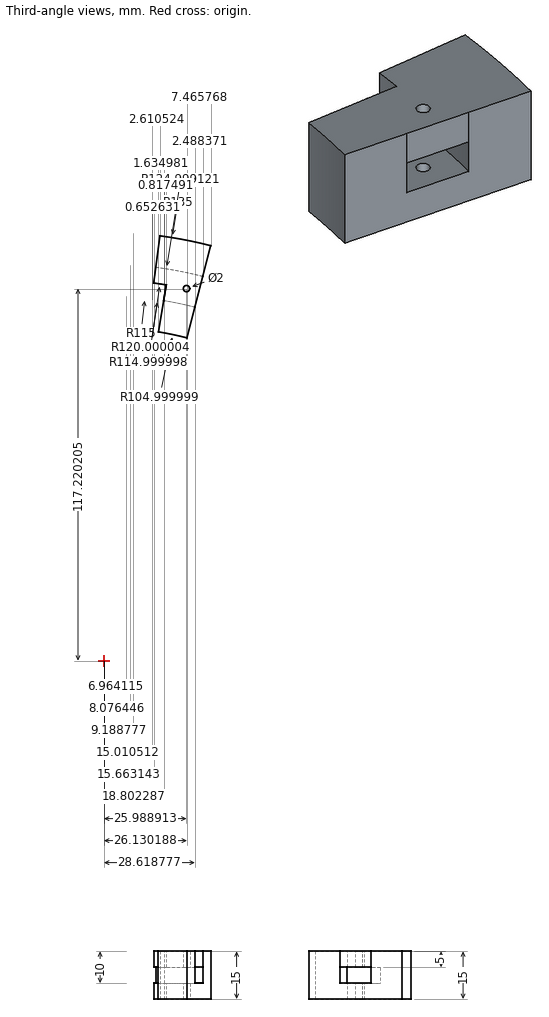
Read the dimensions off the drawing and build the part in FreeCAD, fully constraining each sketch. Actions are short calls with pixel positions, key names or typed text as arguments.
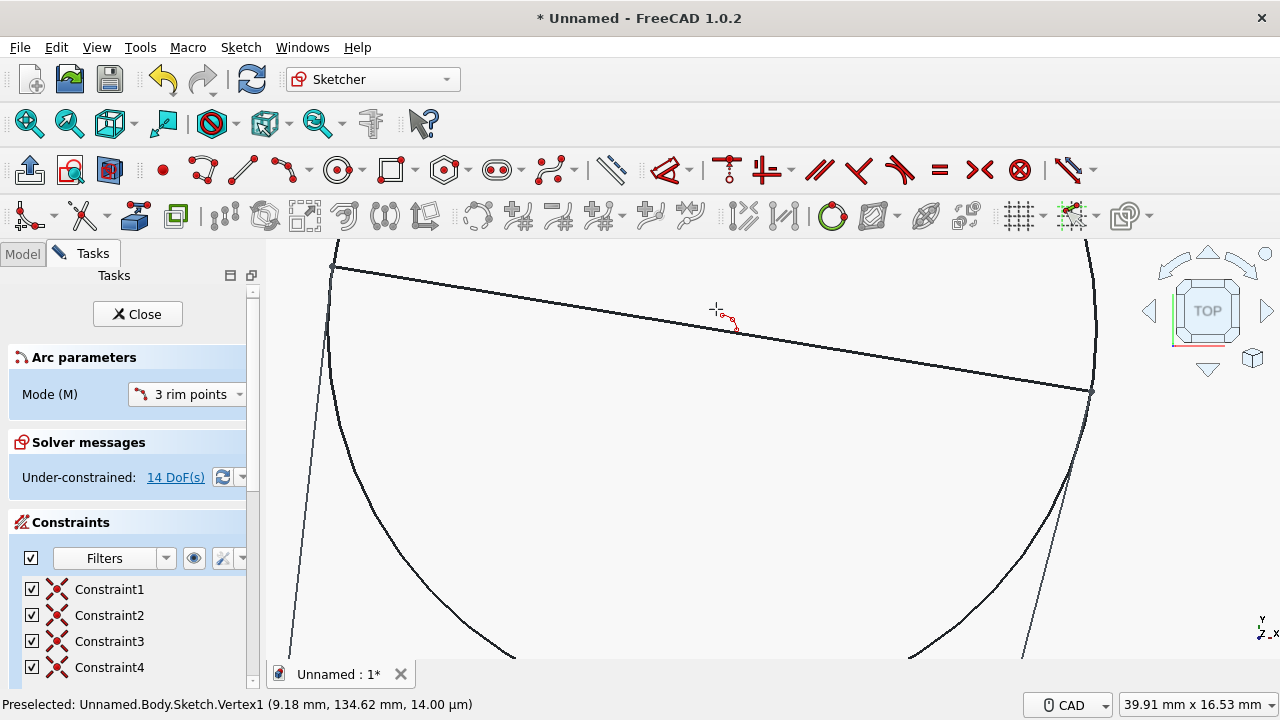
click(714, 308)
key(Escape)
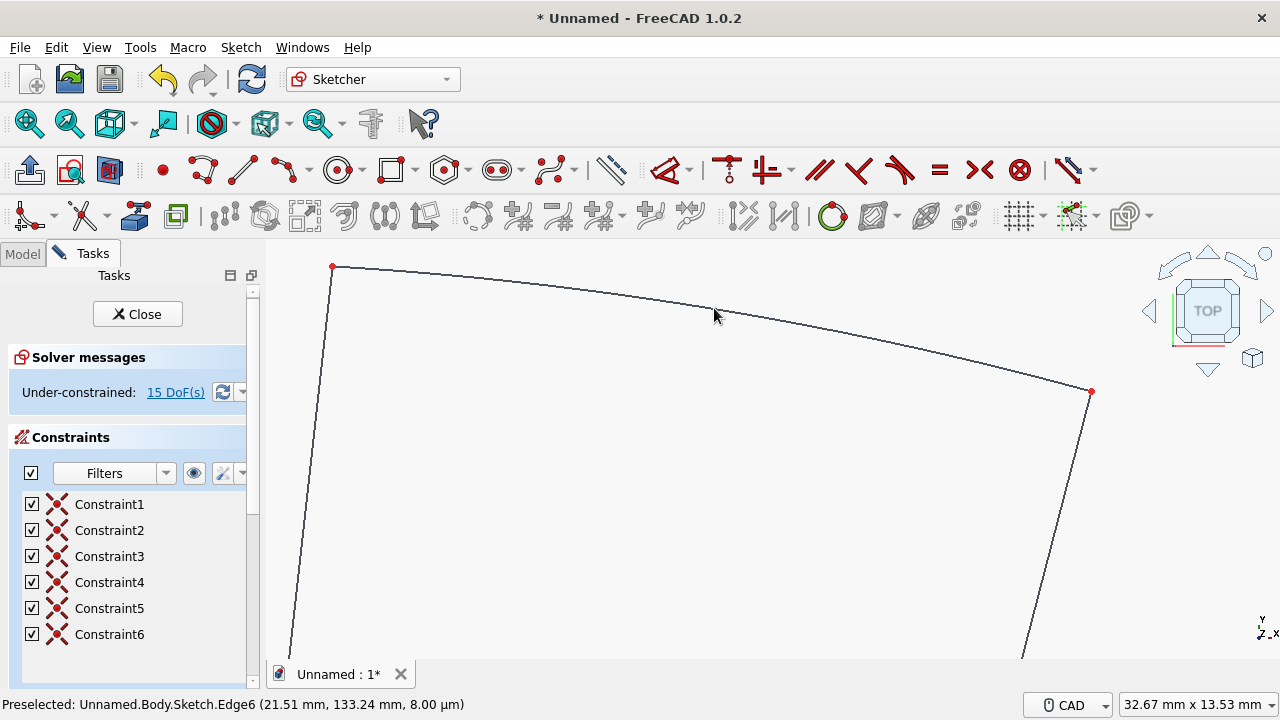
scroll(713, 342, down, 7)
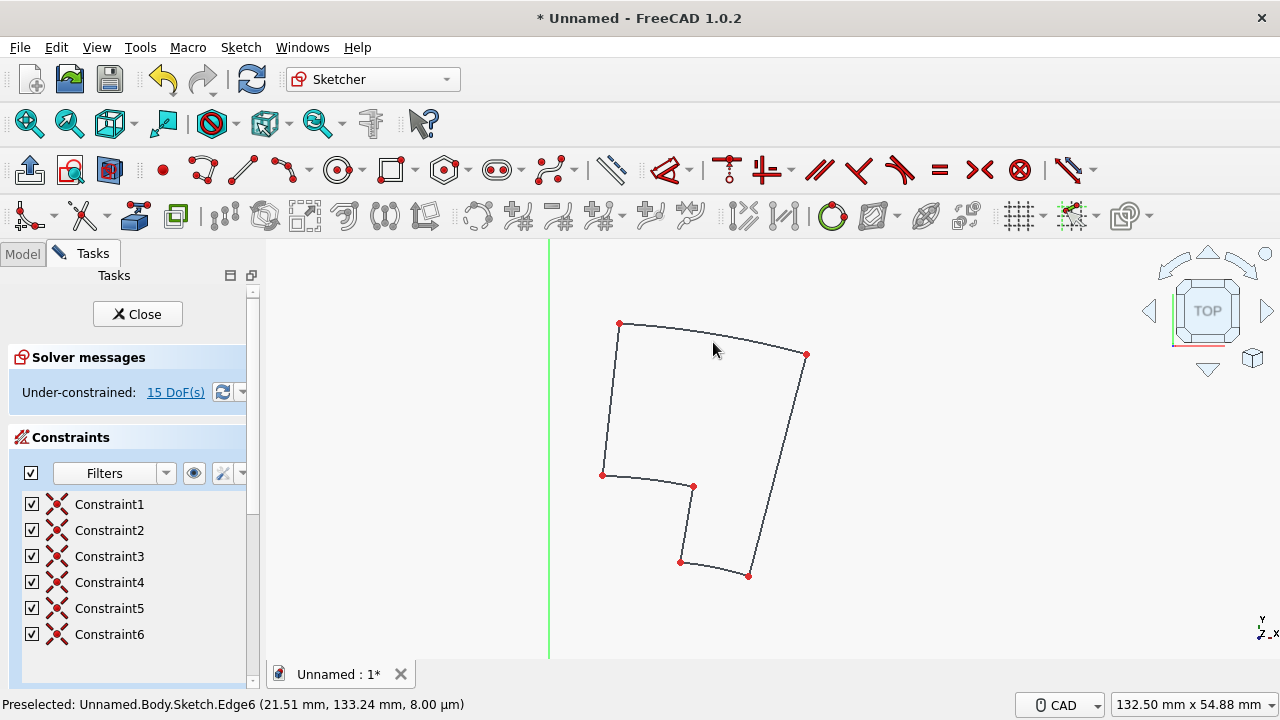
click(666, 482)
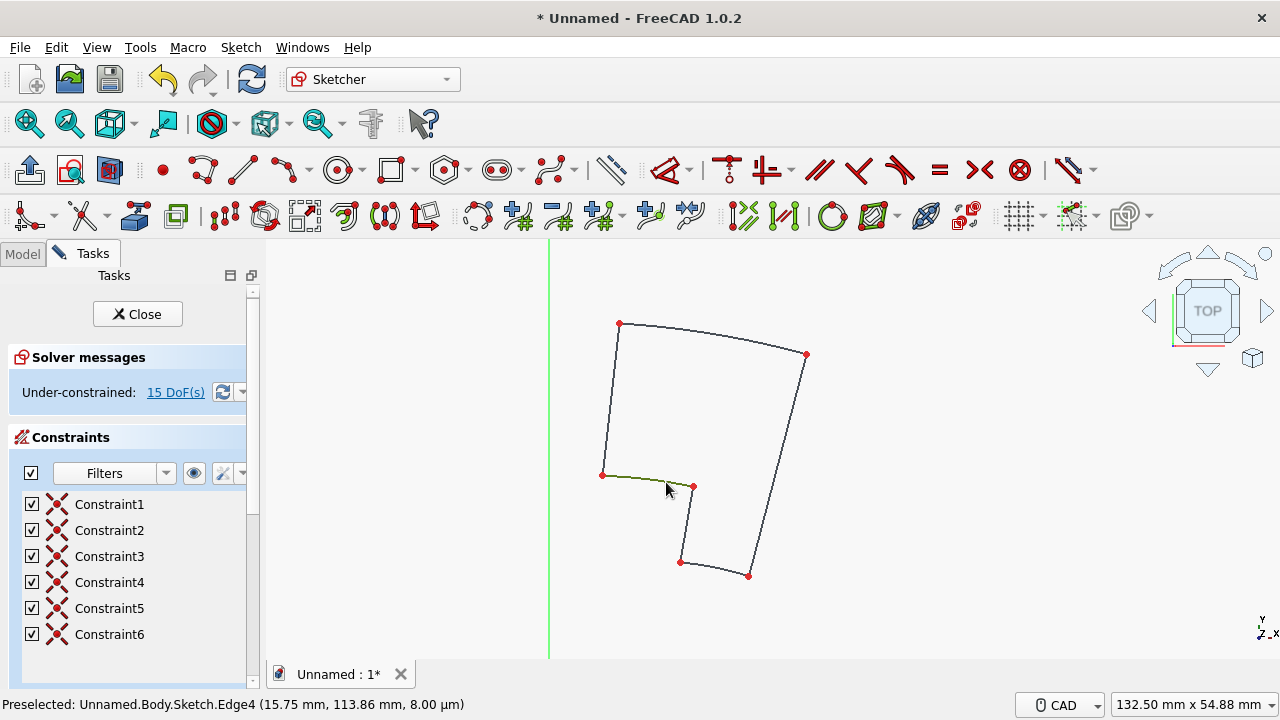
click(729, 571)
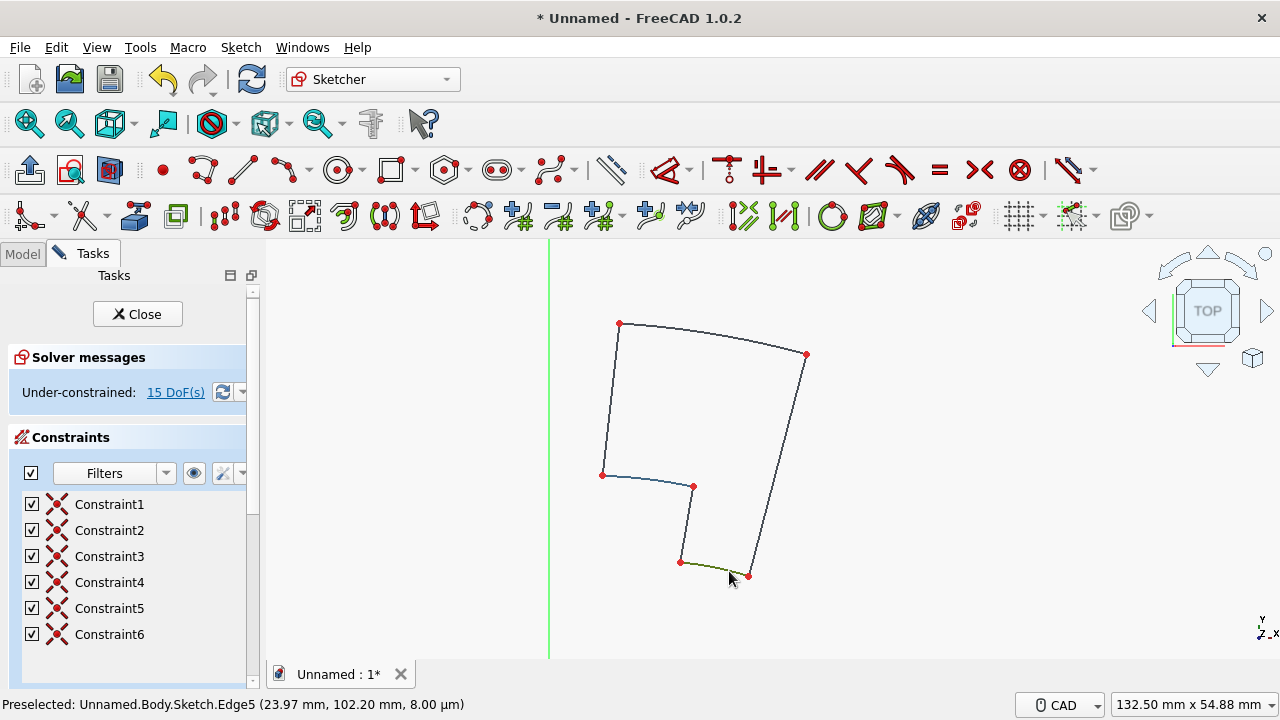
click(728, 170)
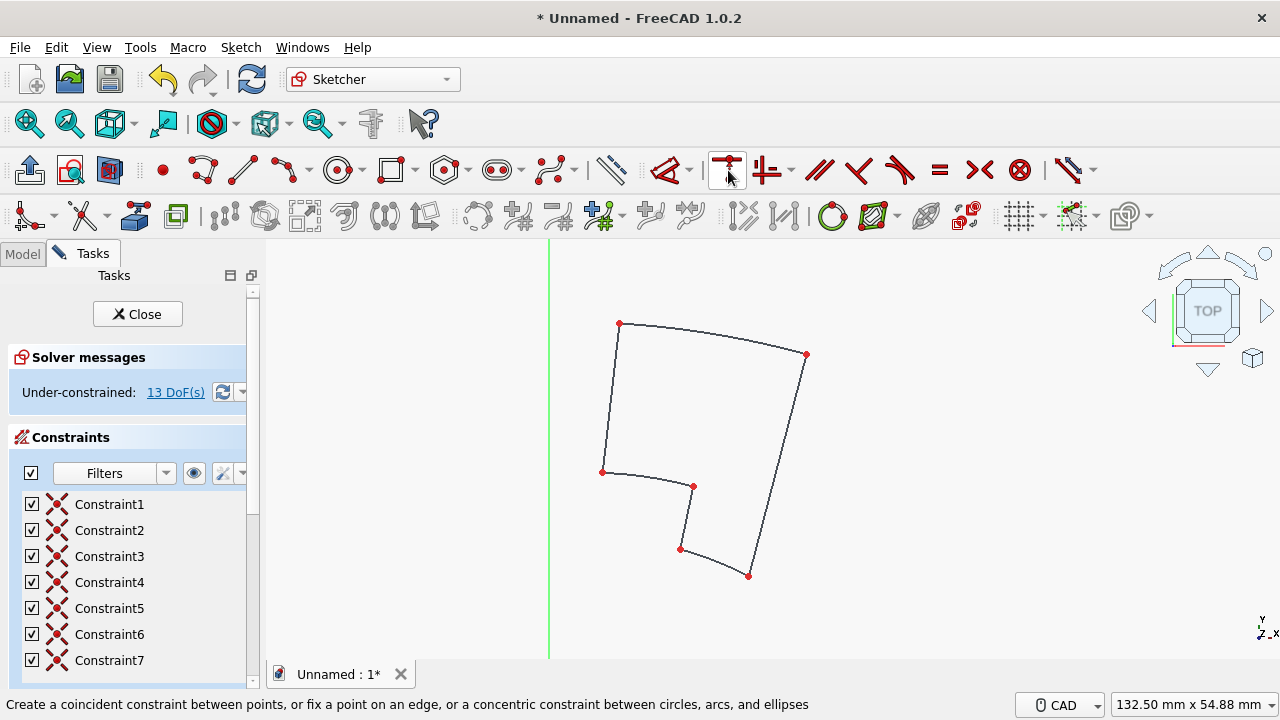
click(666, 480)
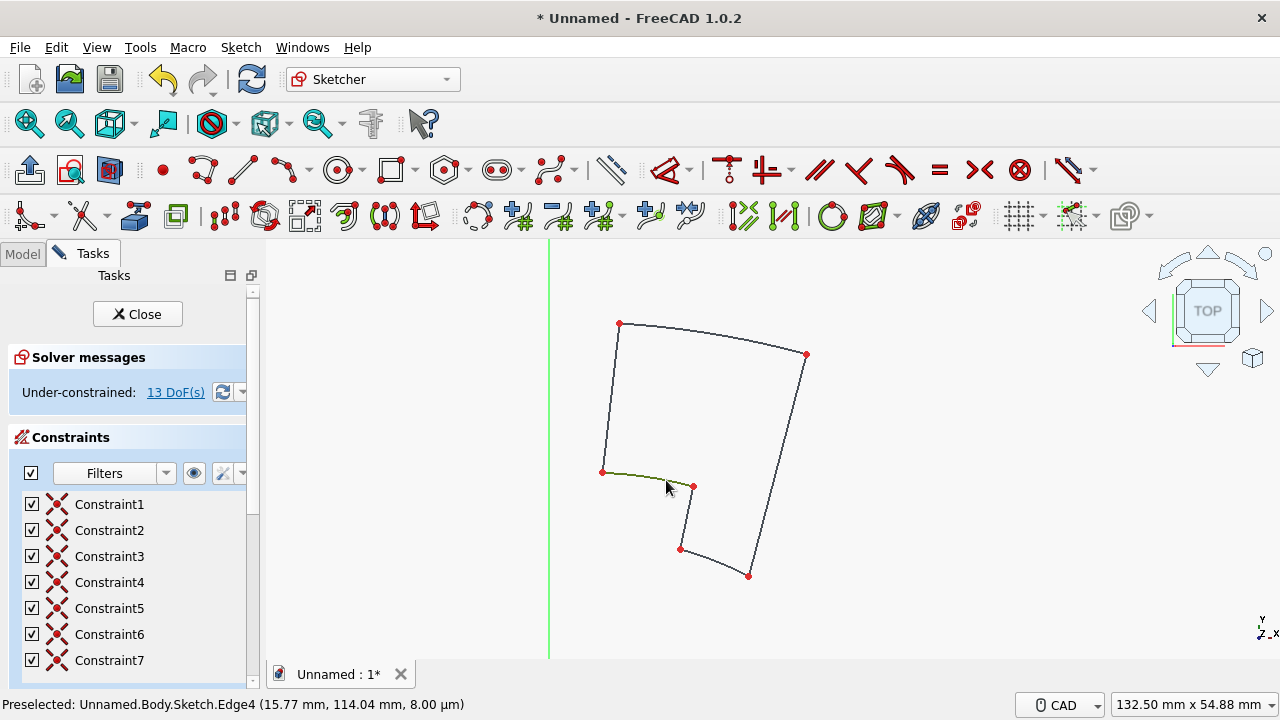
click(751, 341)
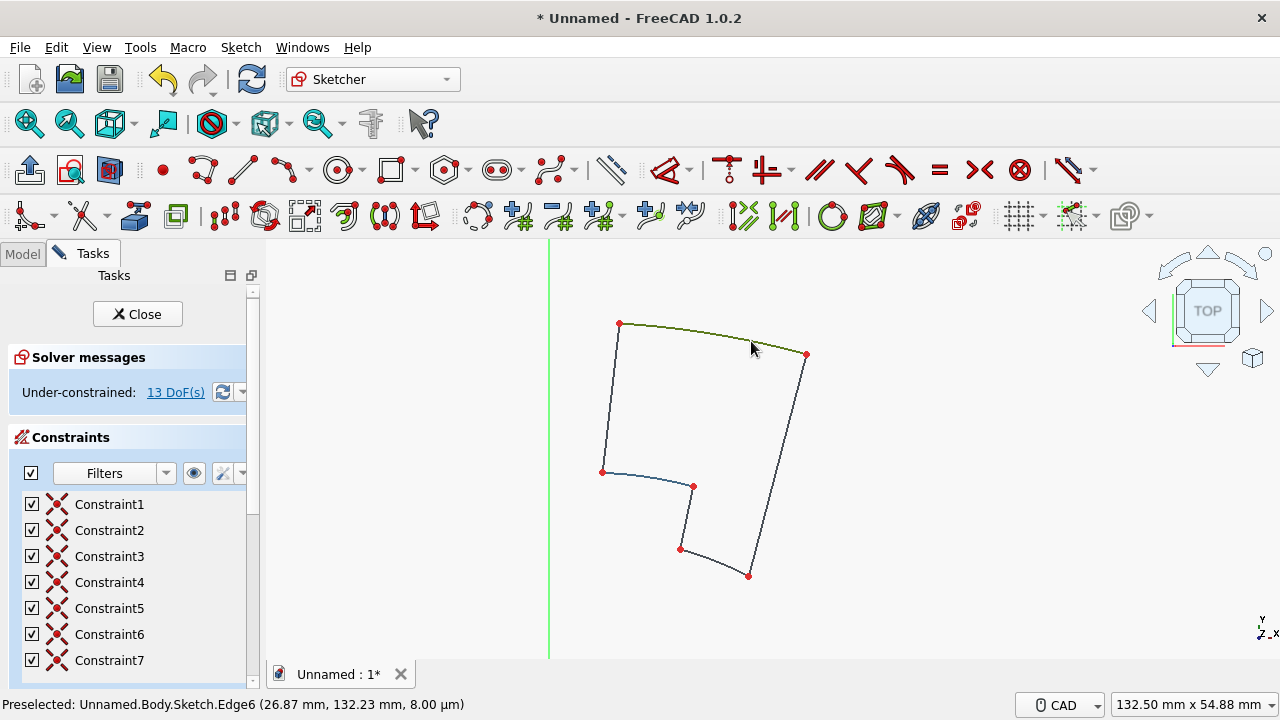
click(728, 170)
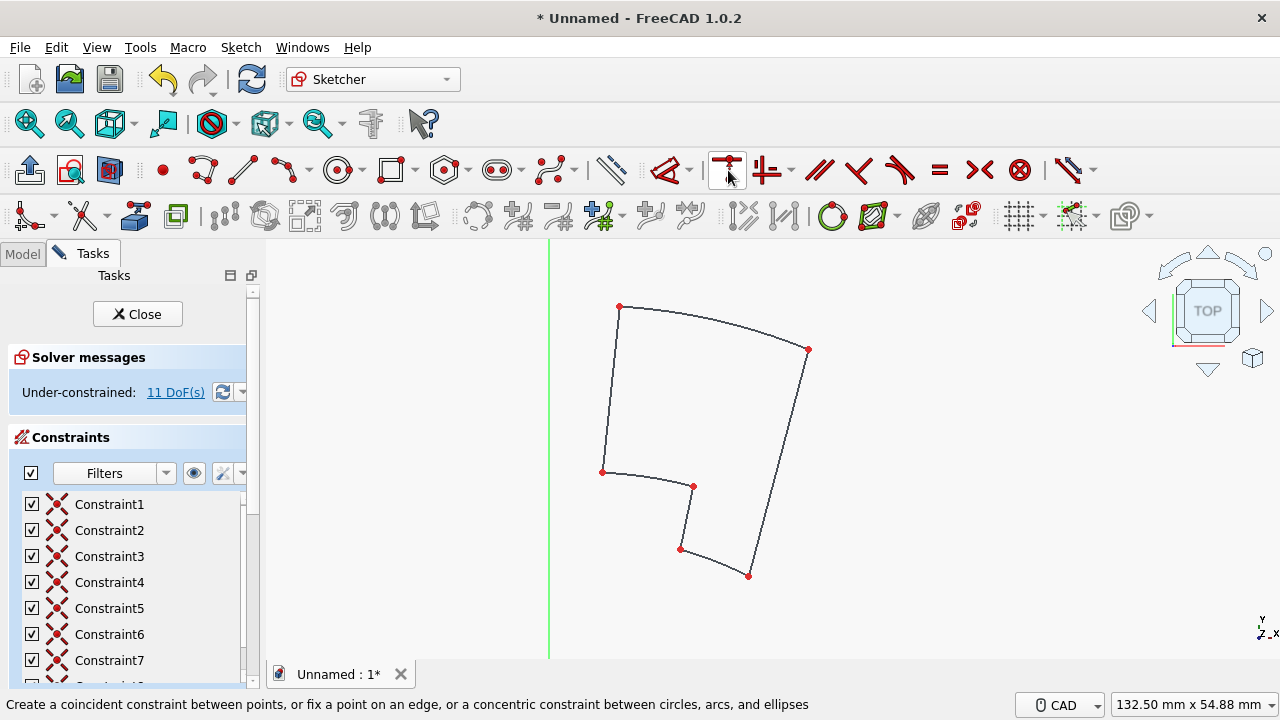
scroll(712, 330, down, 6)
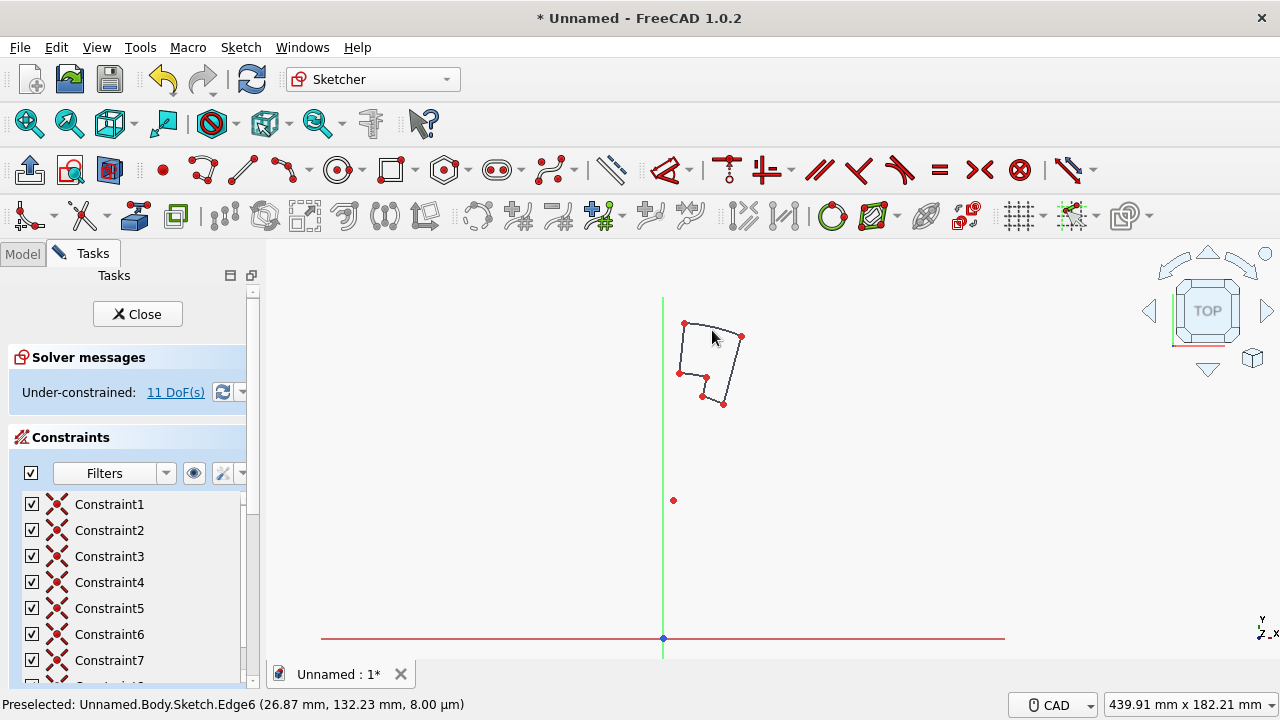
drag(653, 491, 684, 648)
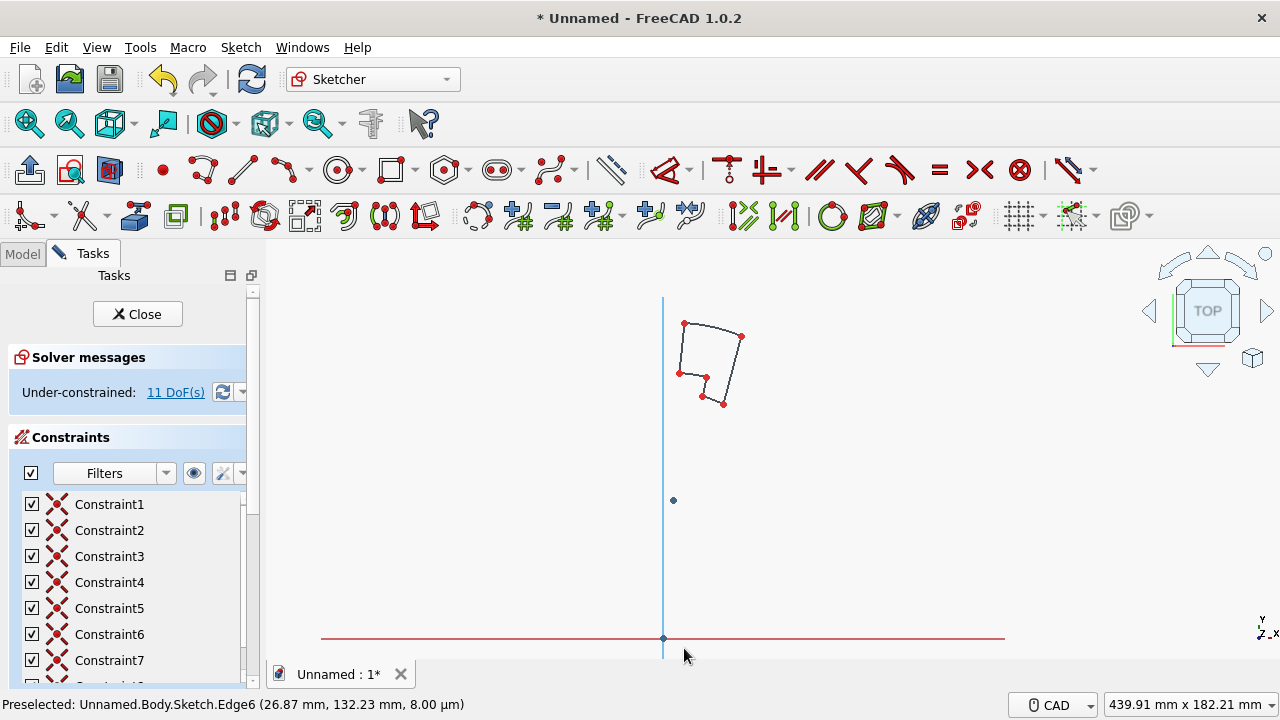
key(c)